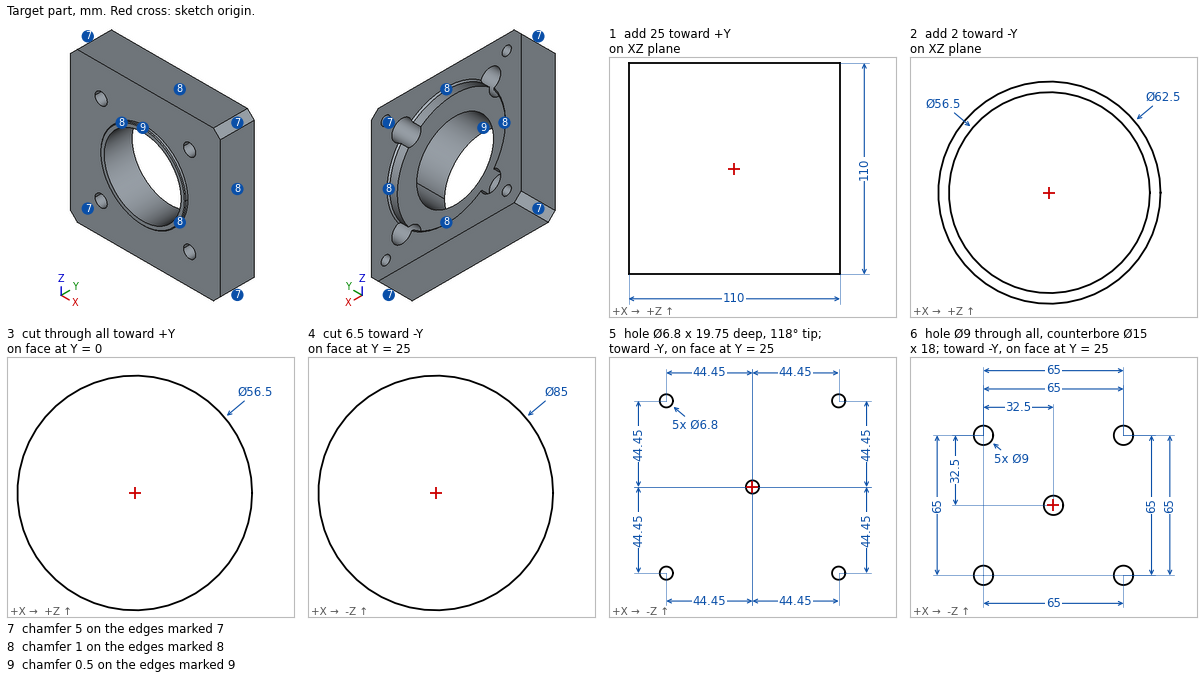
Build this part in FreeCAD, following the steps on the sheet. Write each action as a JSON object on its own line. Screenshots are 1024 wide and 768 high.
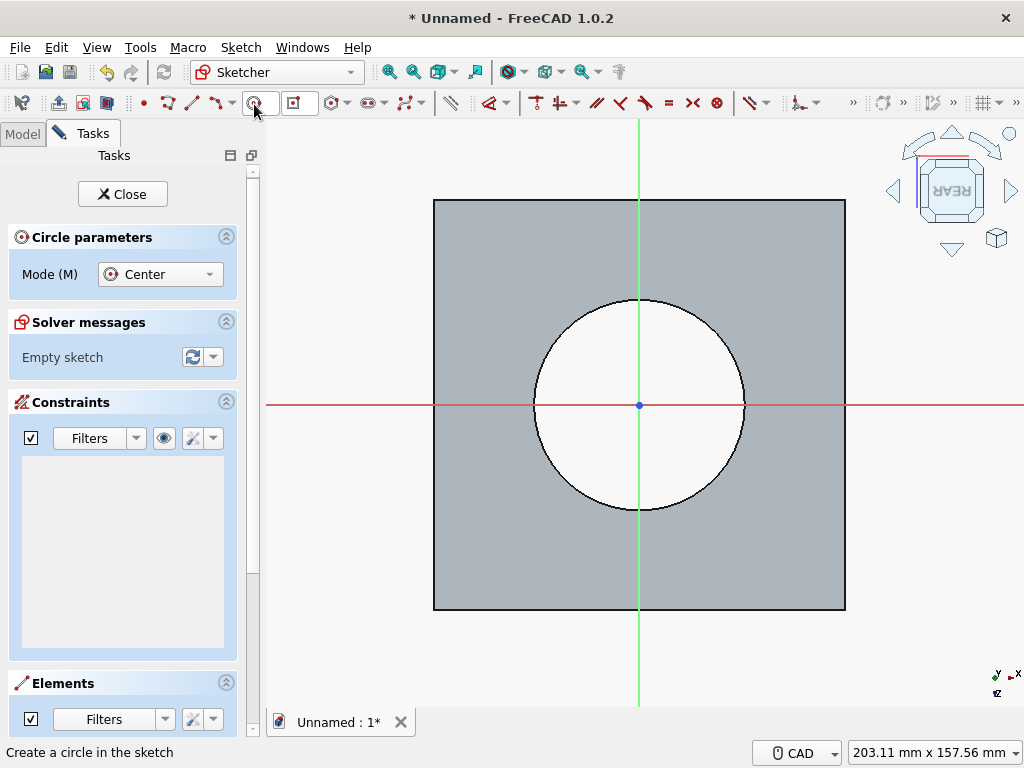
{"action": "left_click", "coordinate": [639, 405]}
{"action": "left_click", "coordinate": [752, 293]}
{"action": "key", "text": "Escape"}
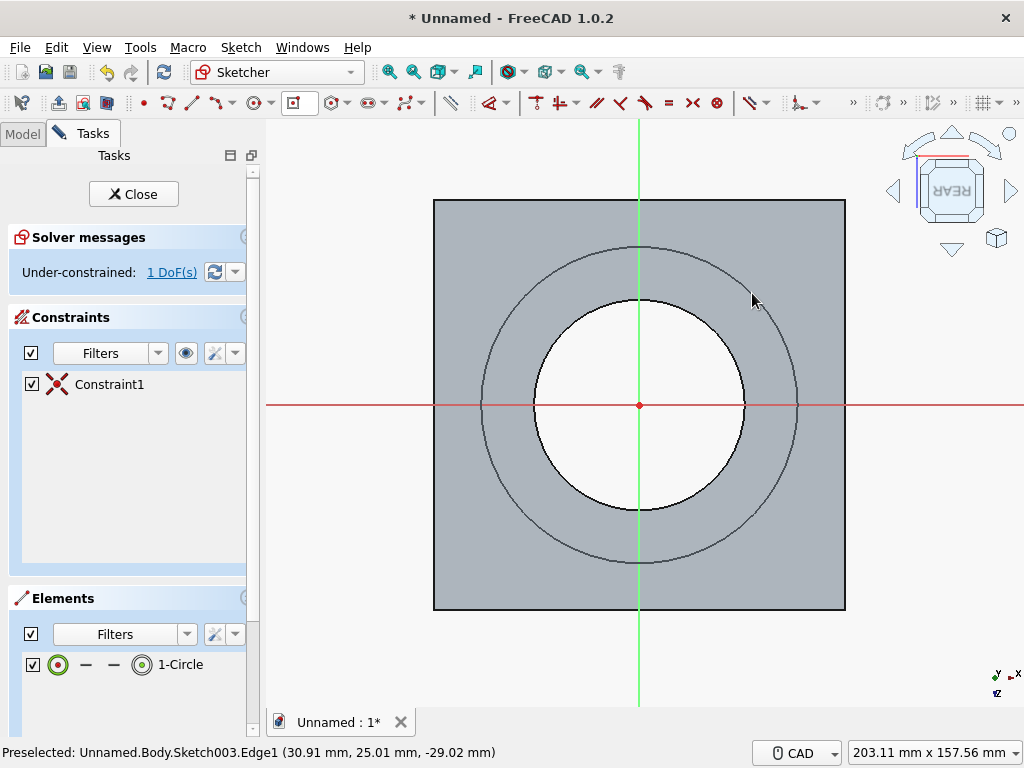
{"action": "left_click", "coordinate": [490, 104]}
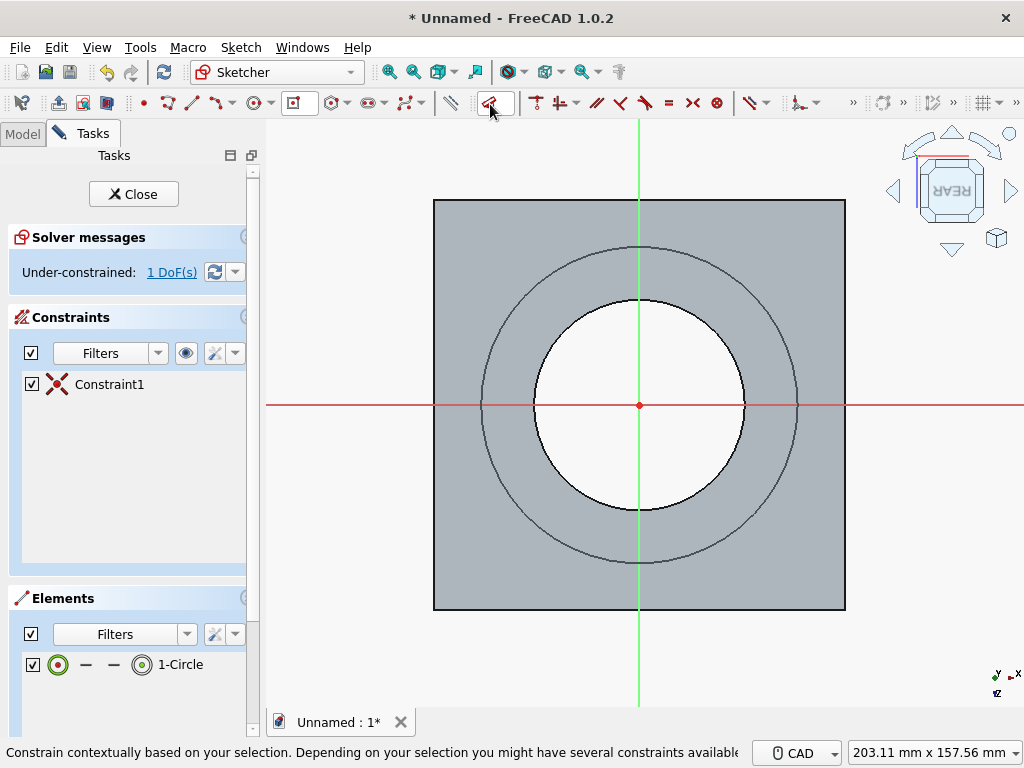
{"action": "left_click", "coordinate": [751, 293]}
{"action": "left_click", "coordinate": [774, 270]}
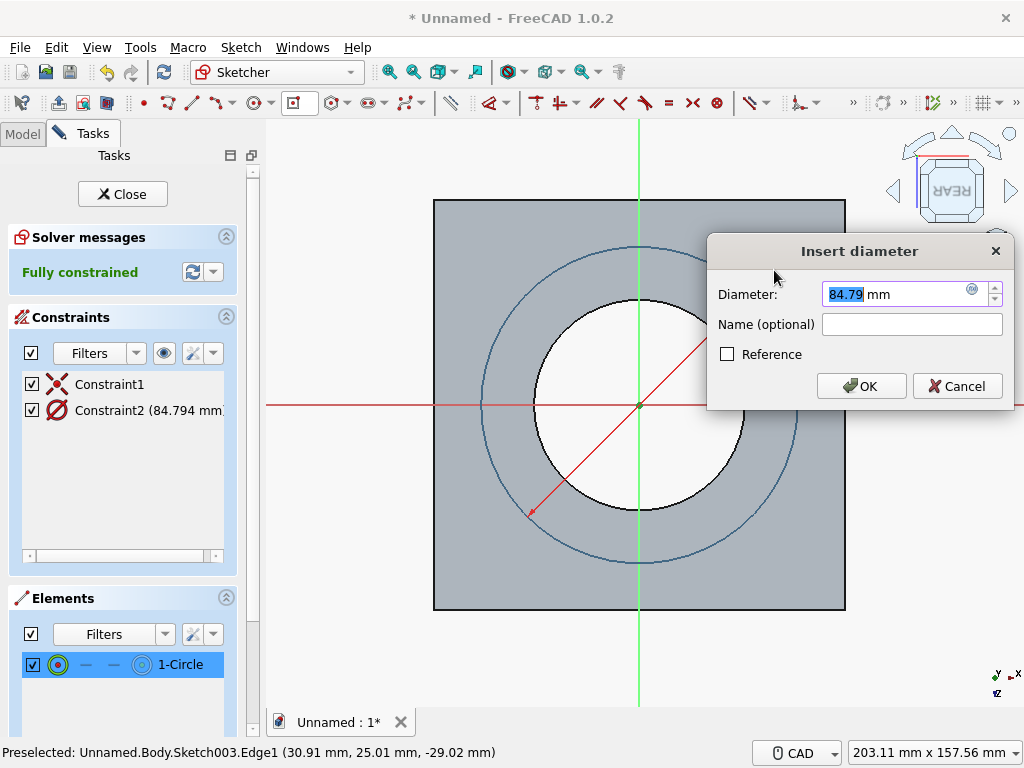
{"action": "type", "text": "85"}
{"action": "key", "text": "Return"}
{"action": "key", "text": "Escape"}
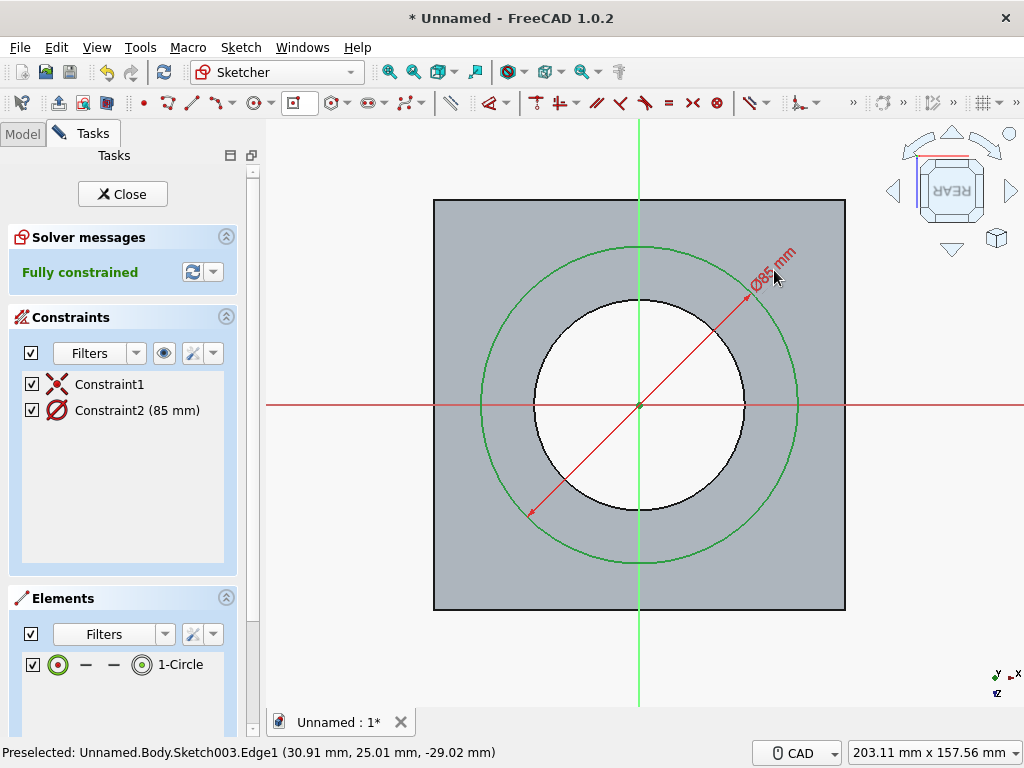
{"action": "left_click", "coordinate": [123, 194]}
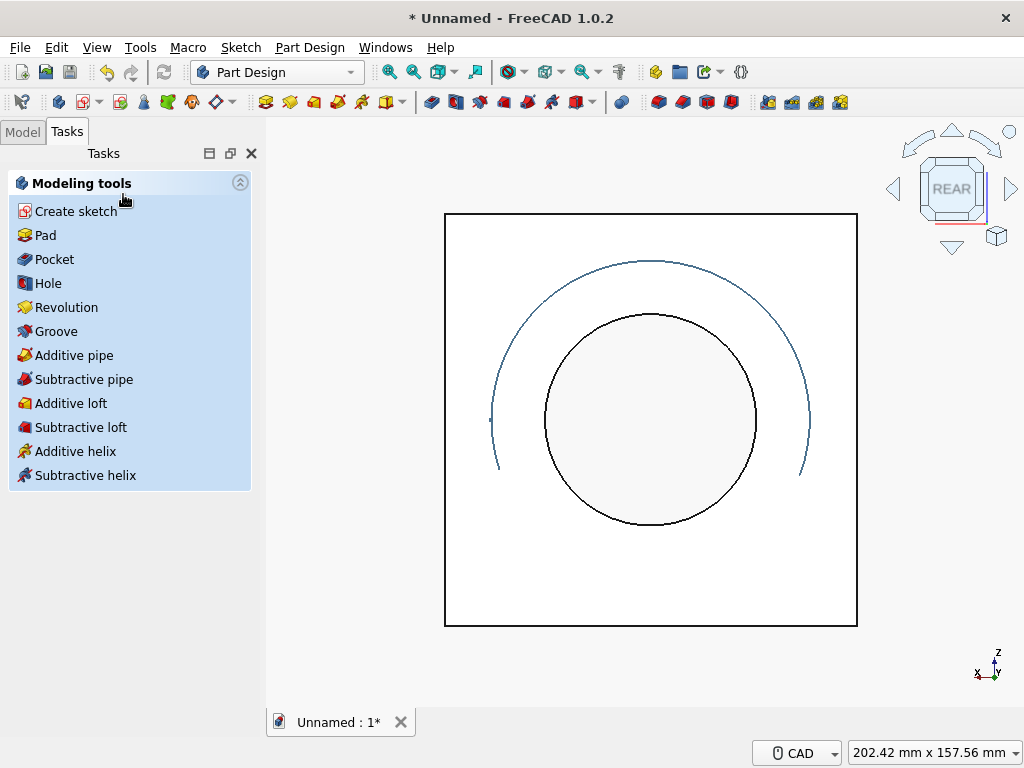
{"action": "left_click", "coordinate": [432, 102]}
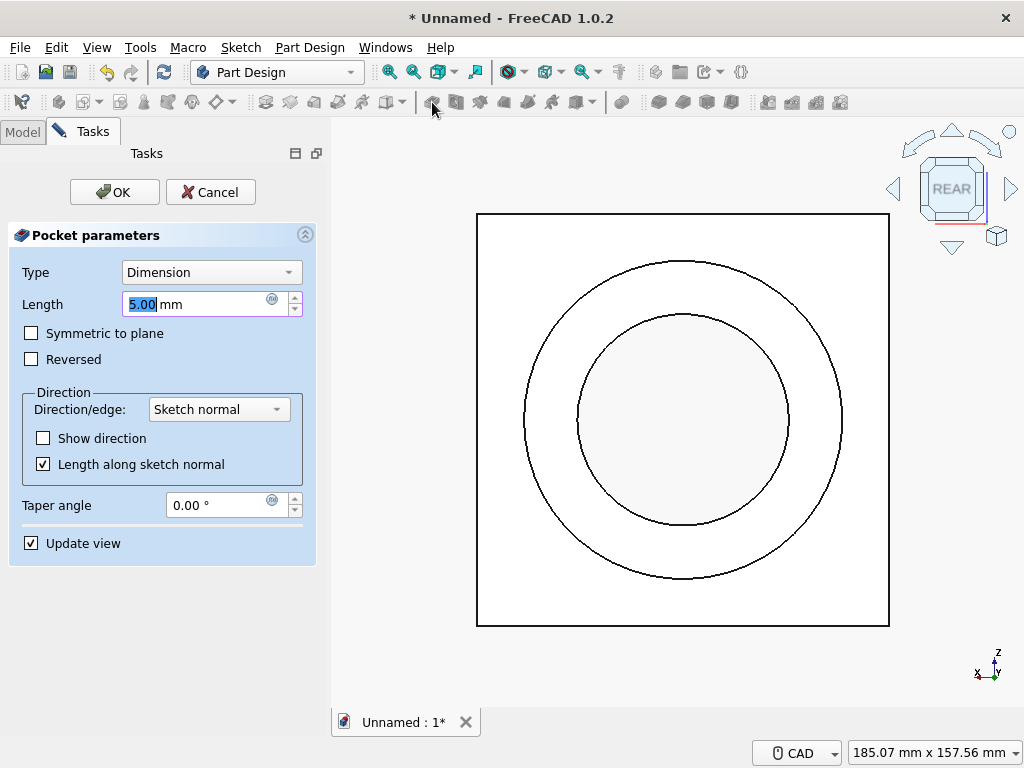
{"action": "type", "text": "6.5"}
{"action": "key", "text": "Tab"}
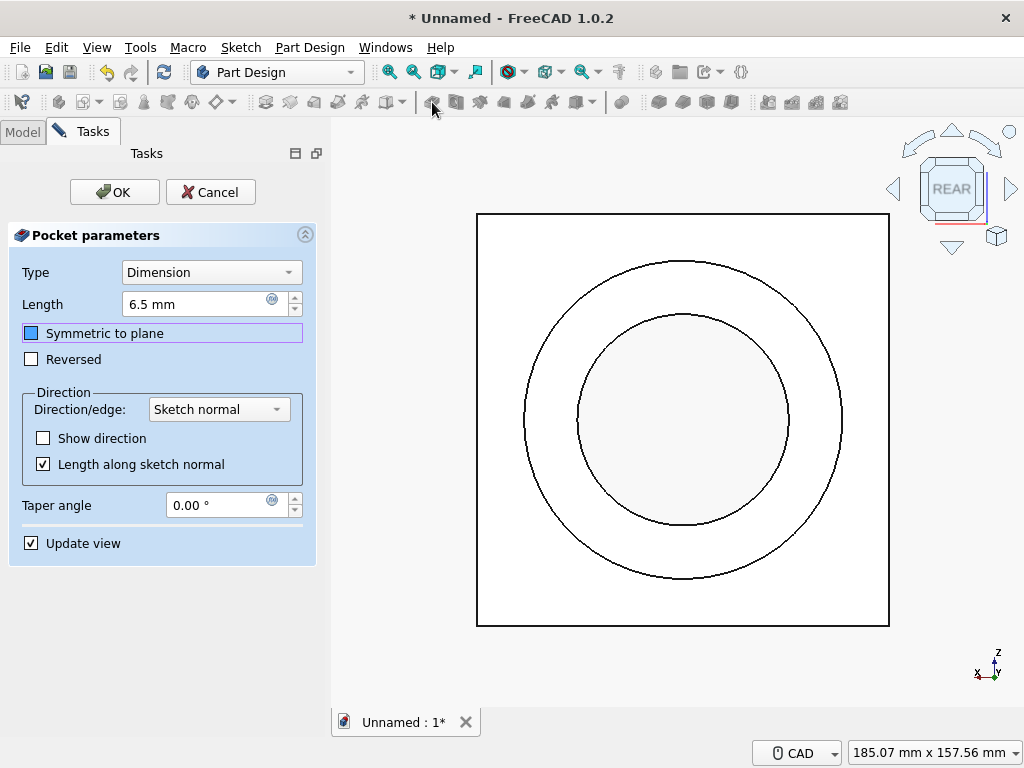
{"action": "left_click", "coordinate": [115, 192]}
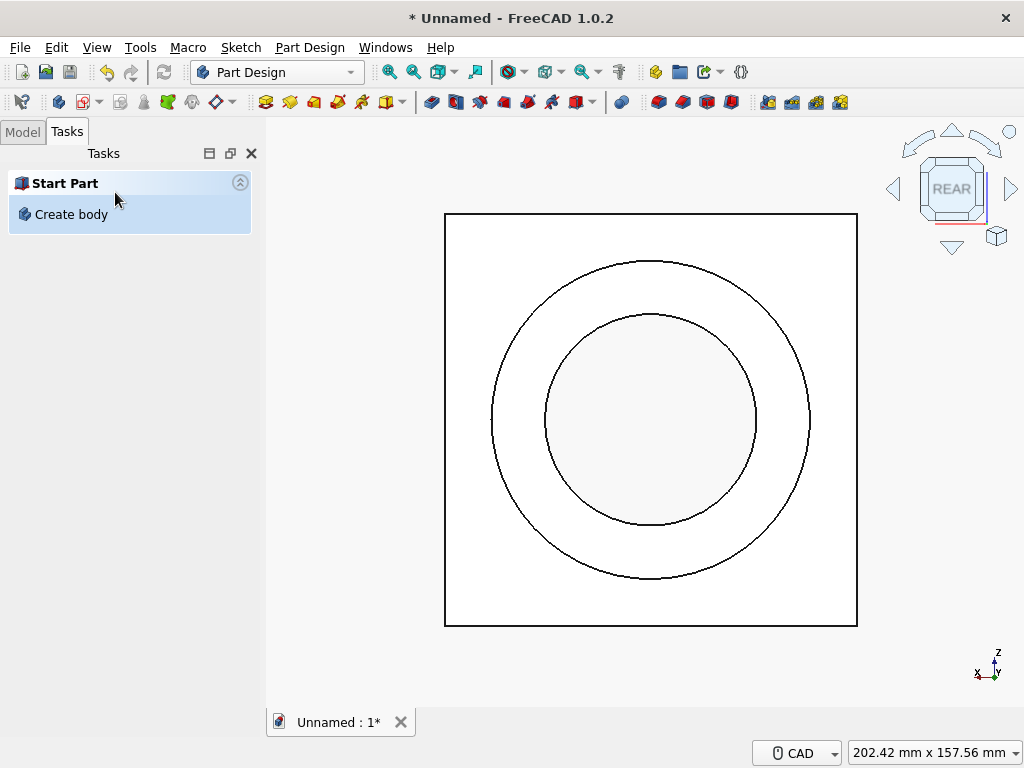
{"action": "left_click", "coordinate": [474, 242]}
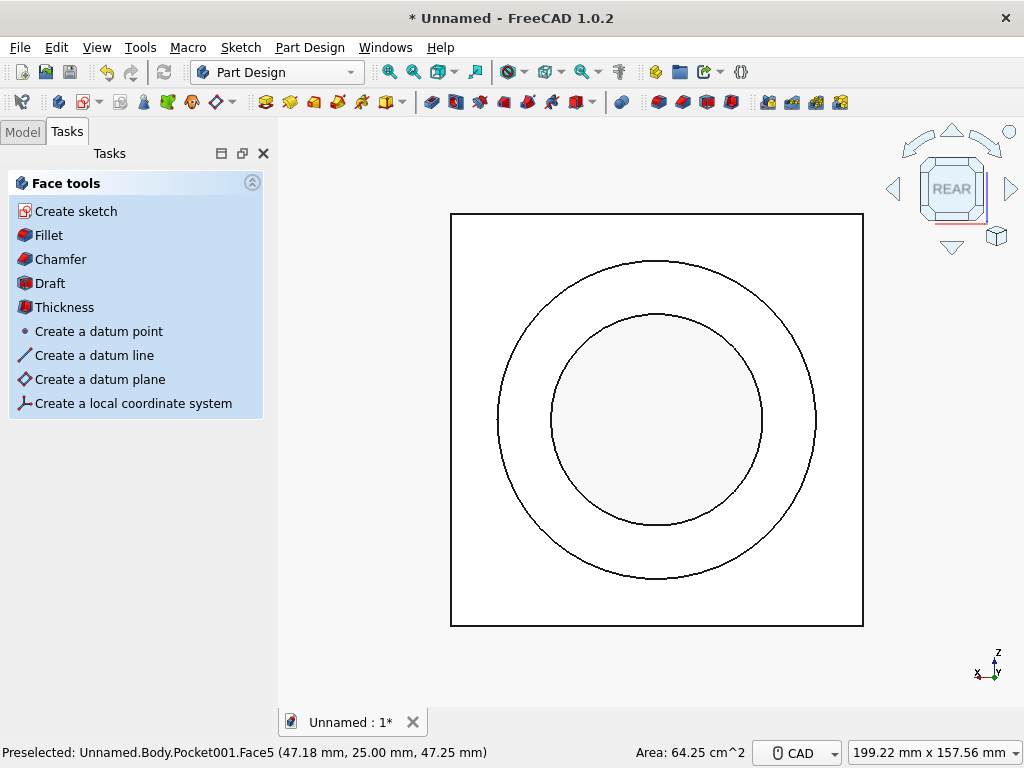
{"action": "left_click", "coordinate": [84, 102]}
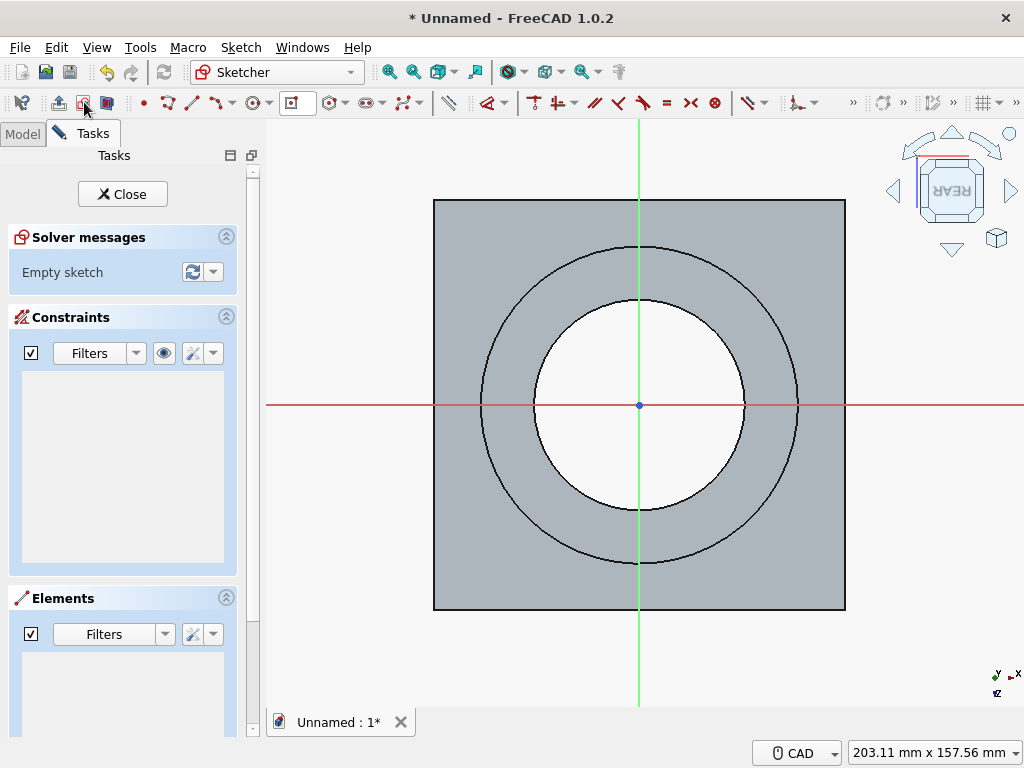
{"action": "left_click", "coordinate": [254, 104]}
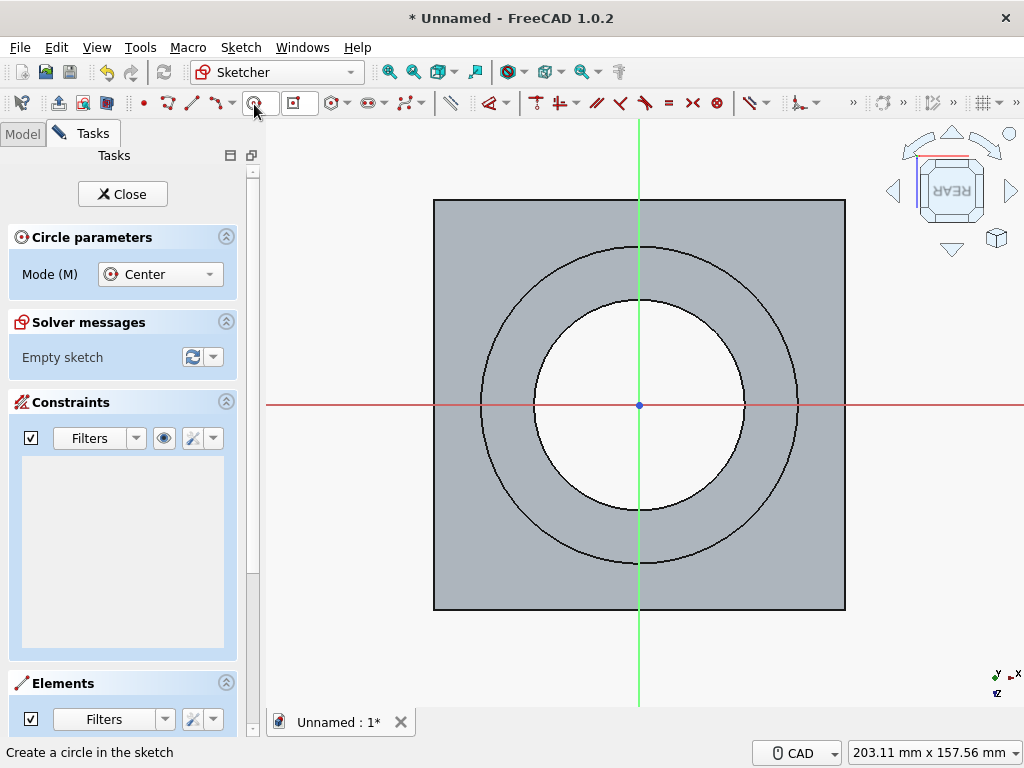
{"action": "scroll", "coordinate": [473, 239], "scroll_direction": "up", "scroll_amount": 3}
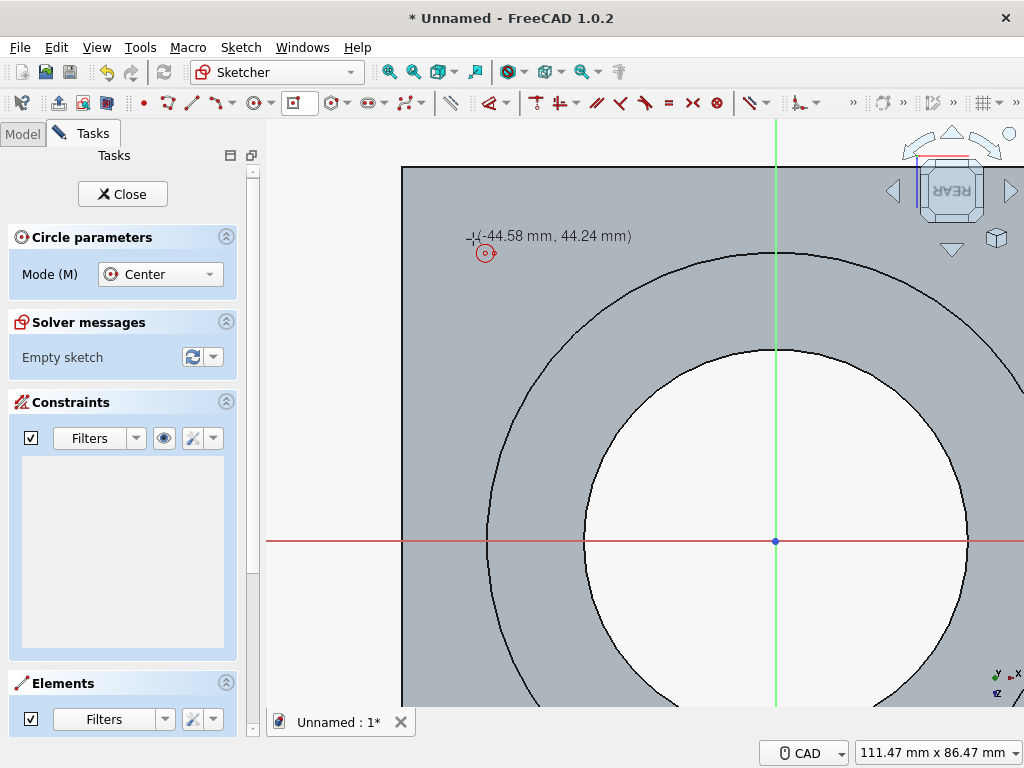
{"action": "left_click", "coordinate": [474, 239]}
{"action": "left_click", "coordinate": [490, 223]}